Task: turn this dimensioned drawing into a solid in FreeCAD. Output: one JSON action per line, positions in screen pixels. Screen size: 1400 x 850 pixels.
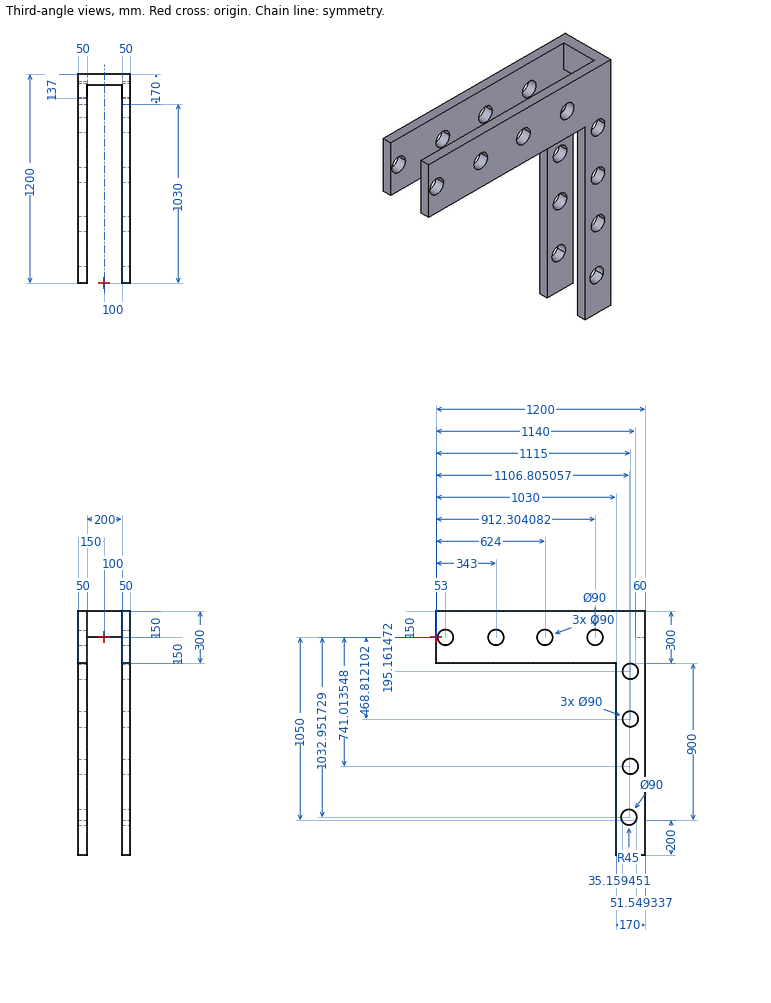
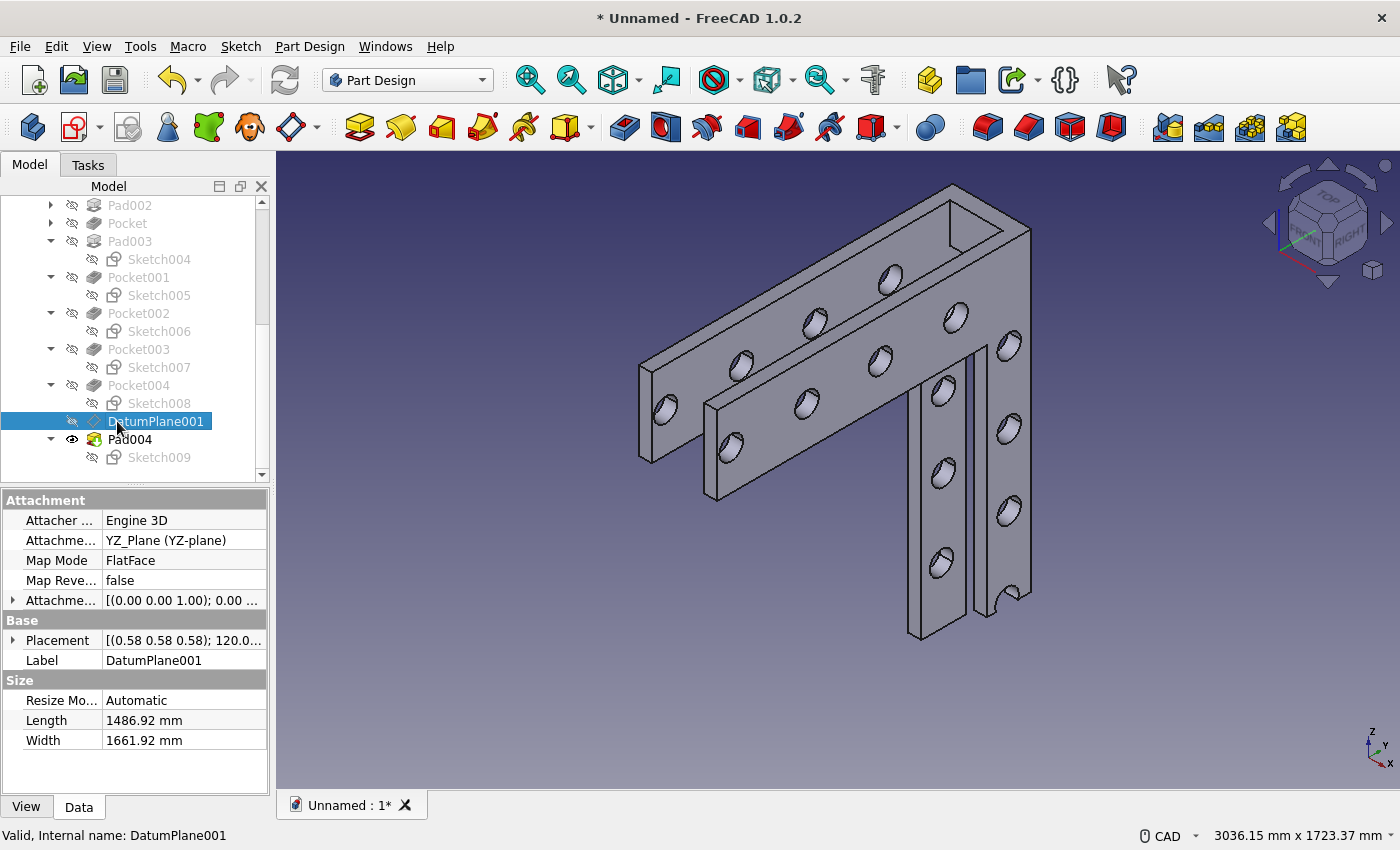
{"action": "left_click", "coordinate": [531, 80]}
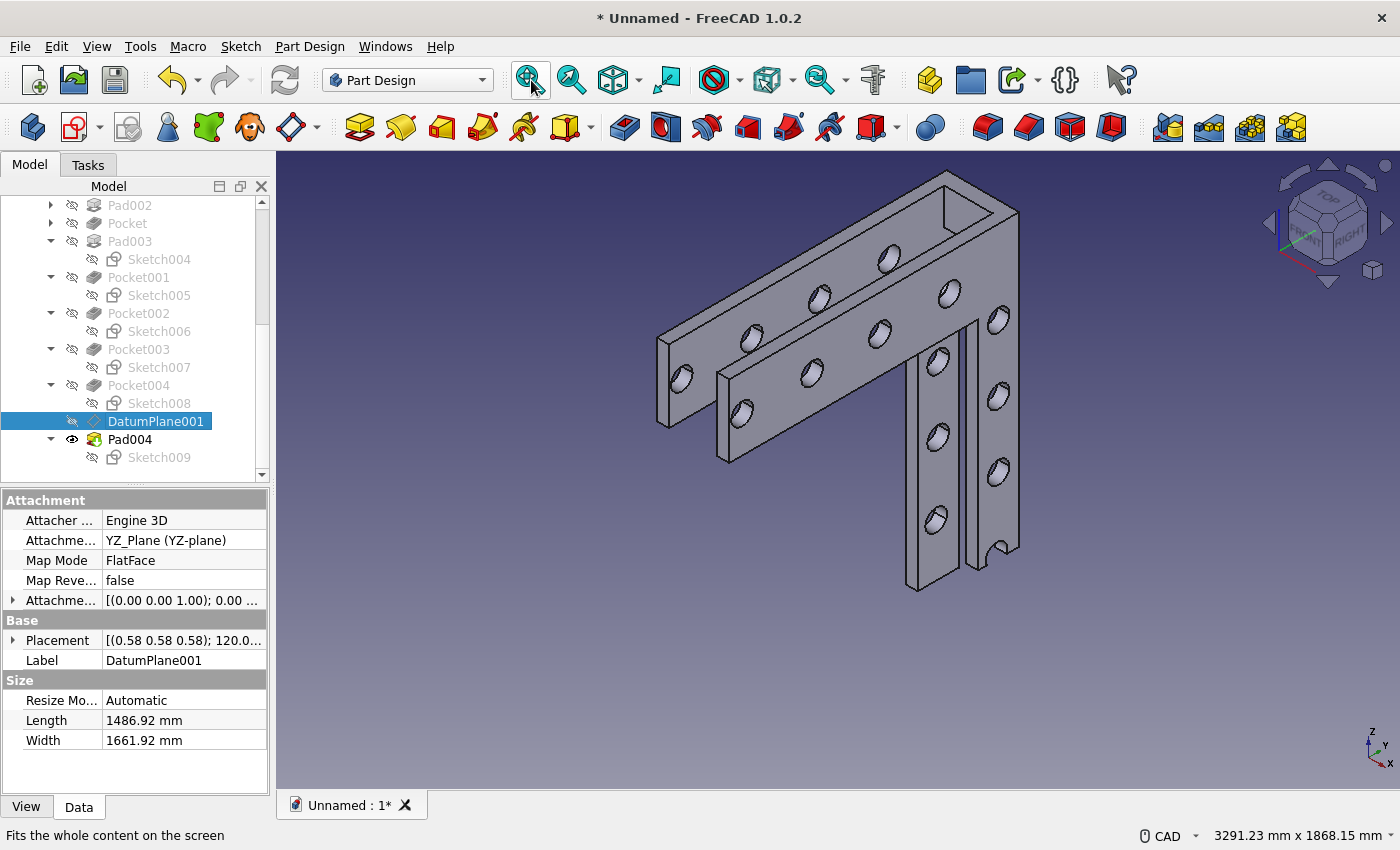
{"action": "left_click", "coordinate": [916, 295]}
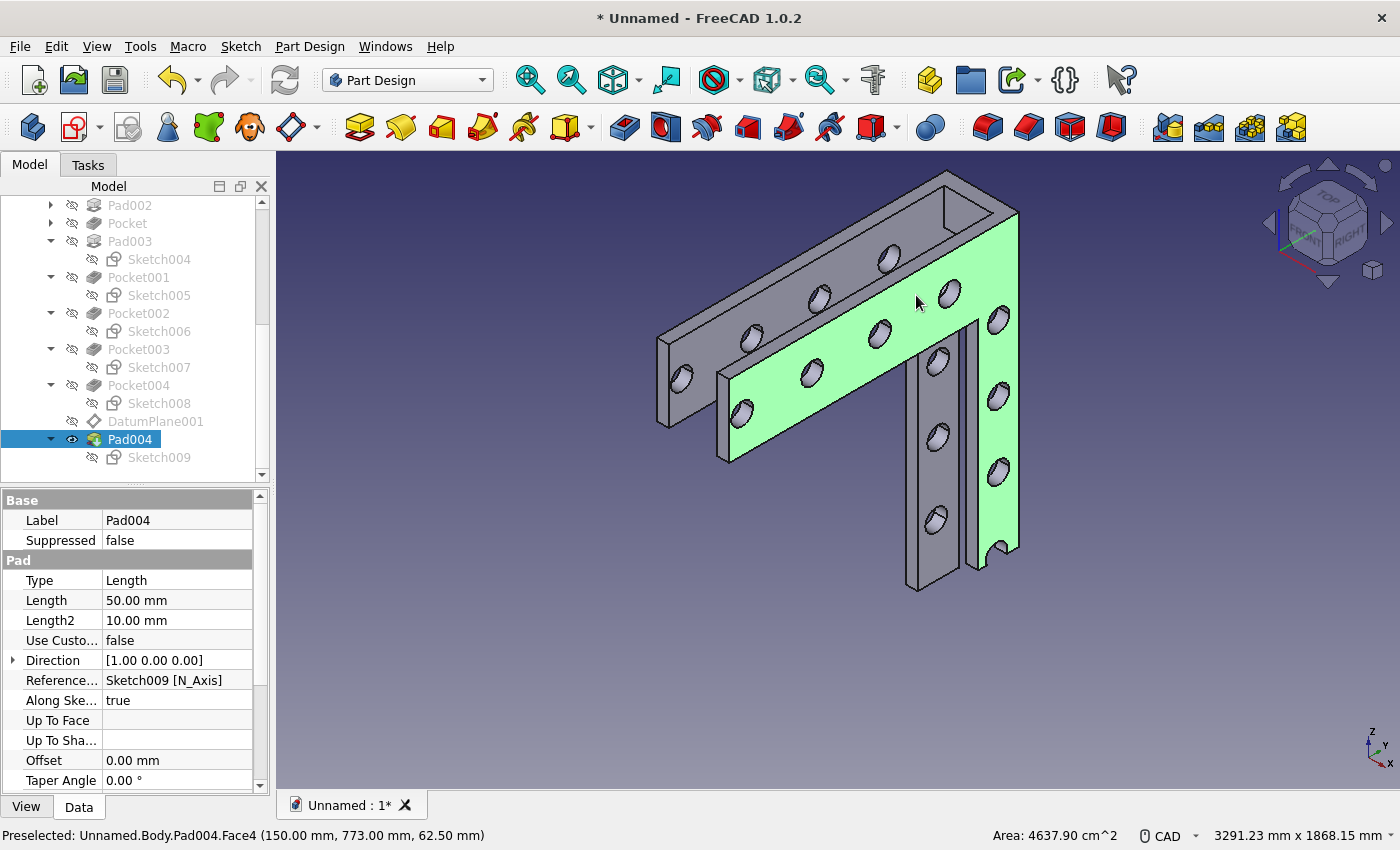
{"action": "left_click", "coordinate": [74, 128]}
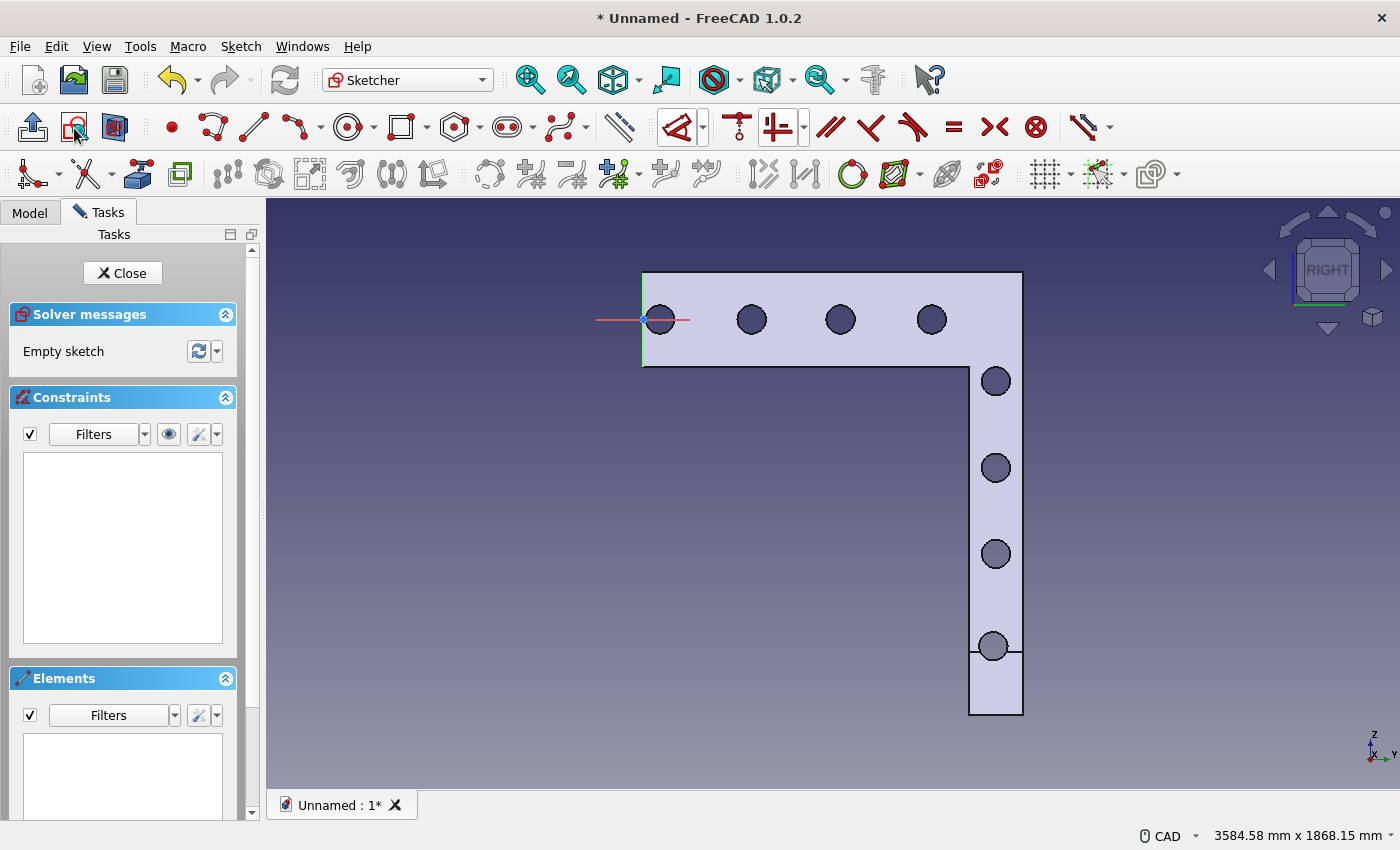
{"action": "scroll", "coordinate": [1042, 721], "scroll_direction": "up", "scroll_amount": 9}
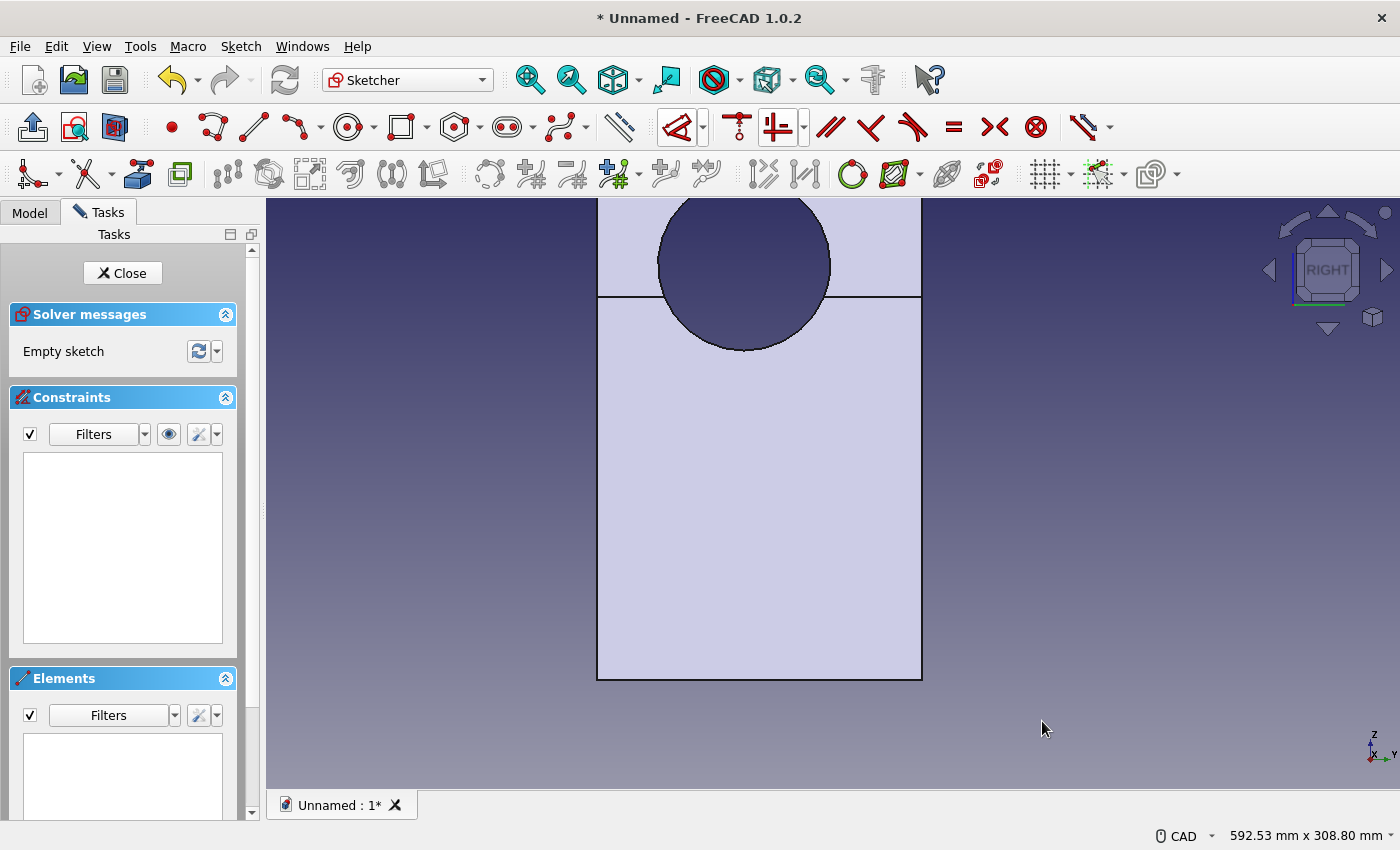
{"action": "left_click", "coordinate": [213, 128]}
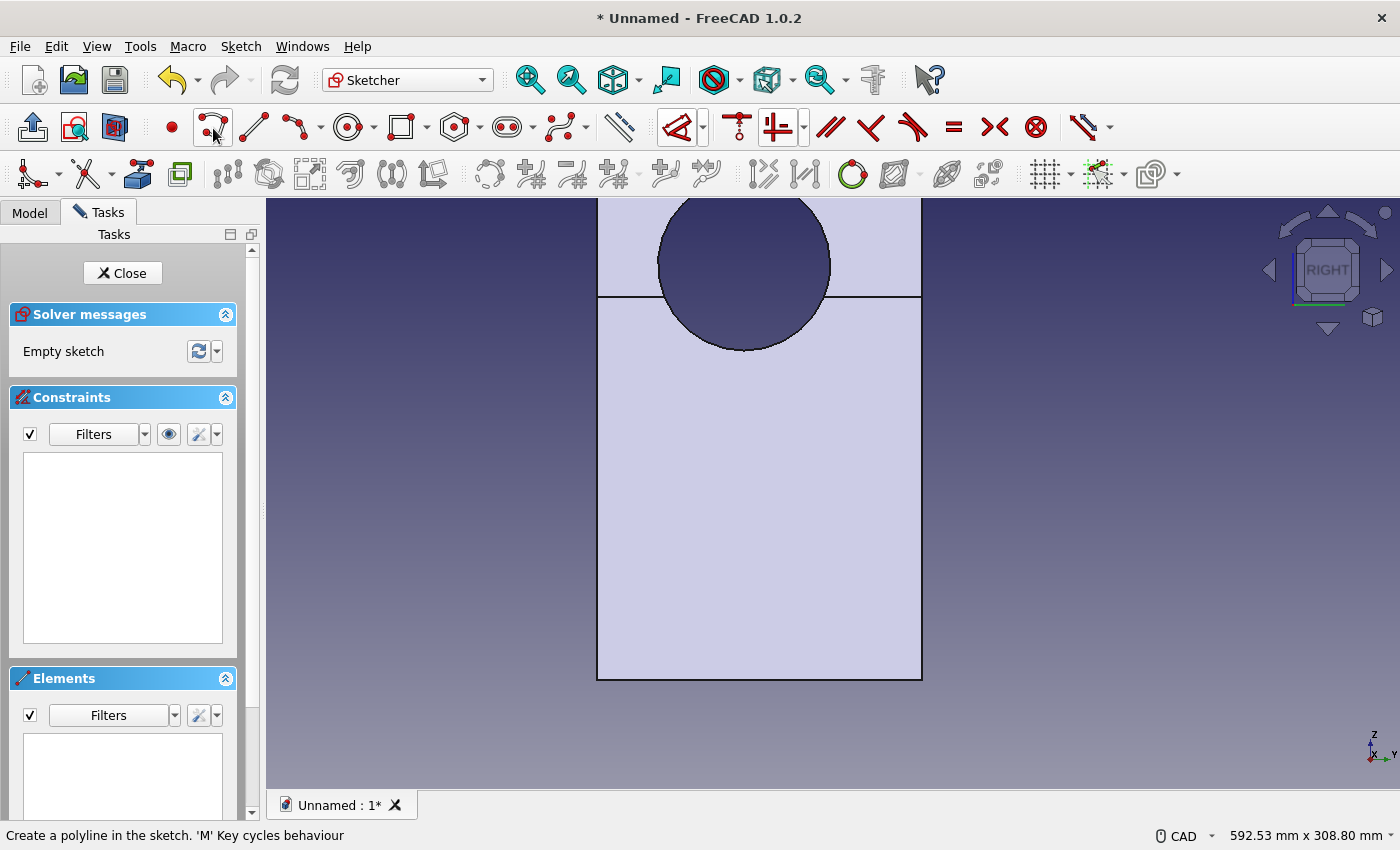
{"action": "left_click", "coordinate": [664, 297]}
{"action": "left_click", "coordinate": [597, 297]}
{"action": "left_click", "coordinate": [597, 680]}
{"action": "left_click", "coordinate": [922, 680]}
{"action": "left_click", "coordinate": [922, 297]}
{"action": "left_click", "coordinate": [824, 297]}
{"action": "right_click", "coordinate": [824, 297]}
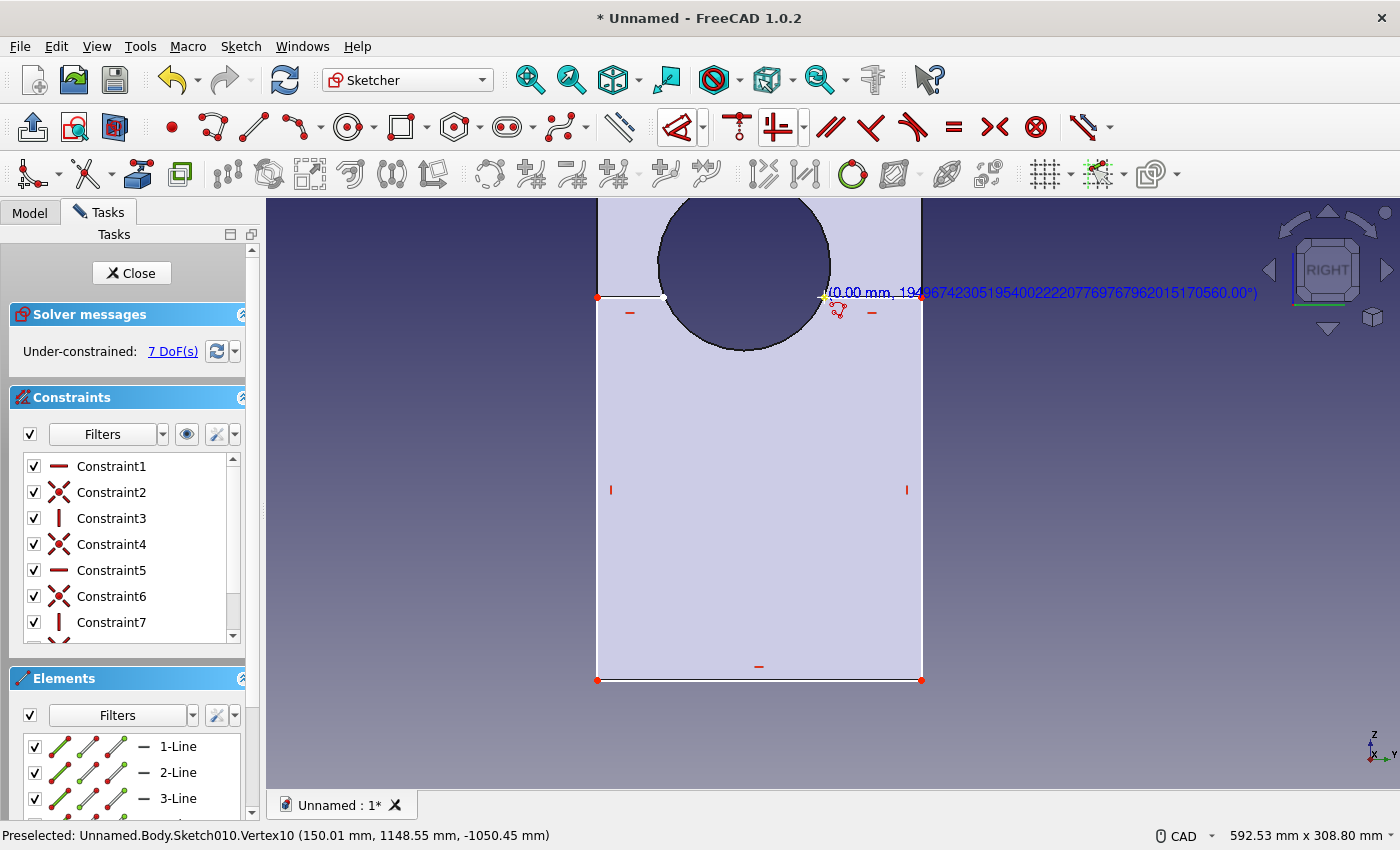
{"action": "left_click", "coordinate": [294, 128]}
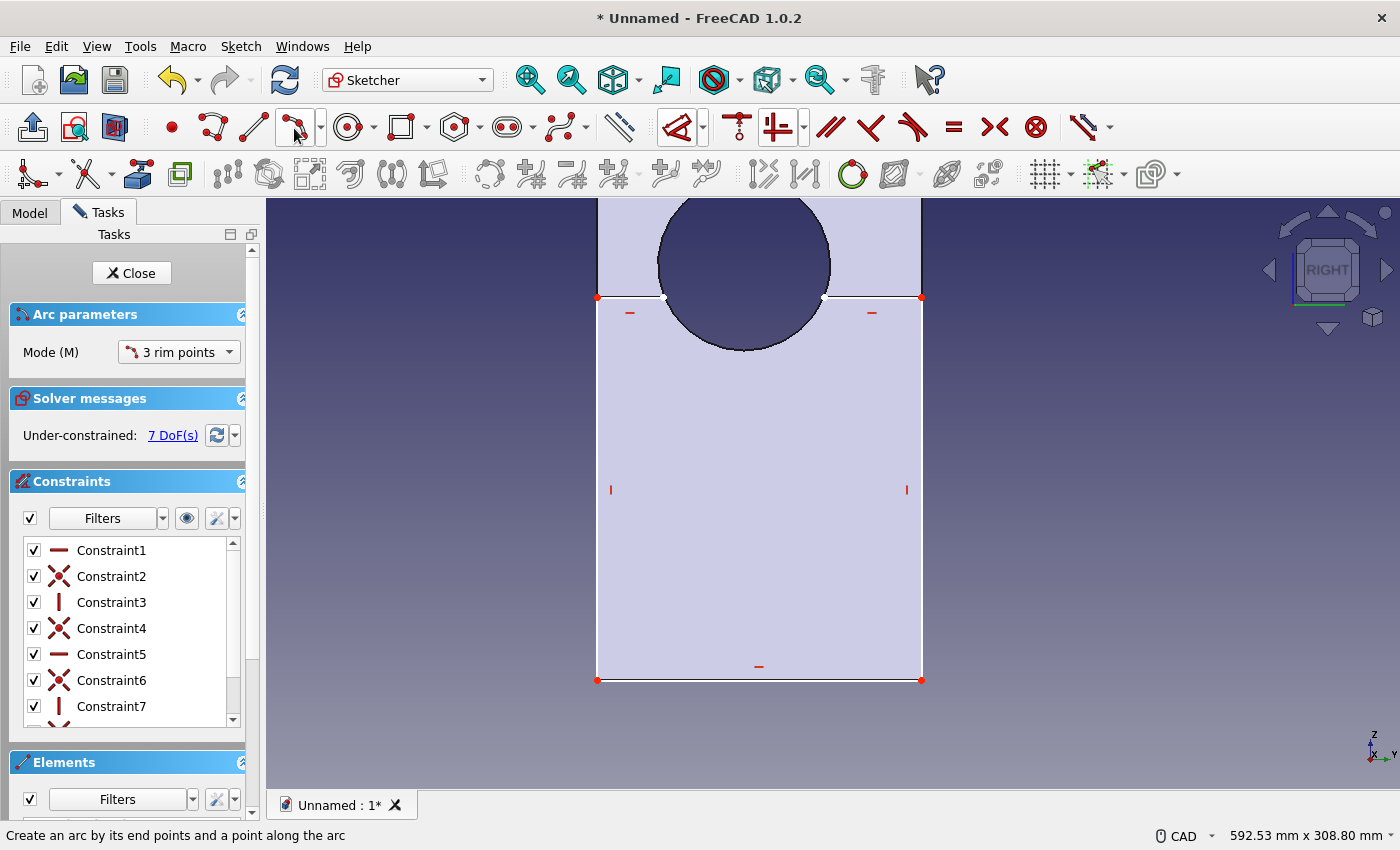
{"action": "left_click", "coordinate": [824, 298]}
{"action": "left_click", "coordinate": [664, 298]}
{"action": "left_click", "coordinate": [744, 351]}
{"action": "key", "text": "Escape"}